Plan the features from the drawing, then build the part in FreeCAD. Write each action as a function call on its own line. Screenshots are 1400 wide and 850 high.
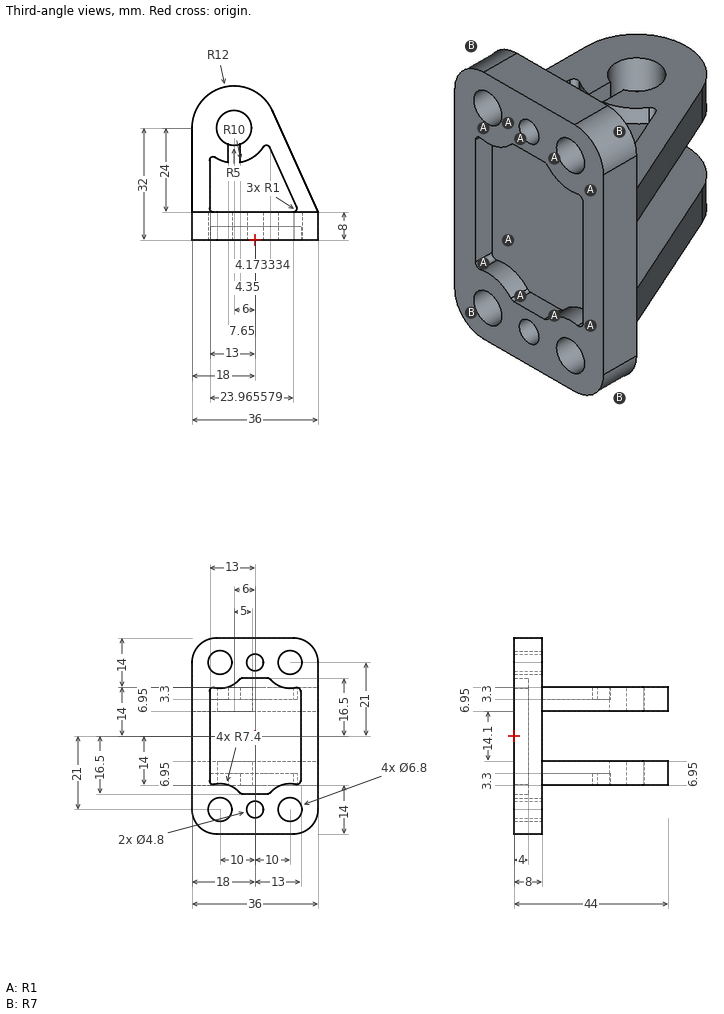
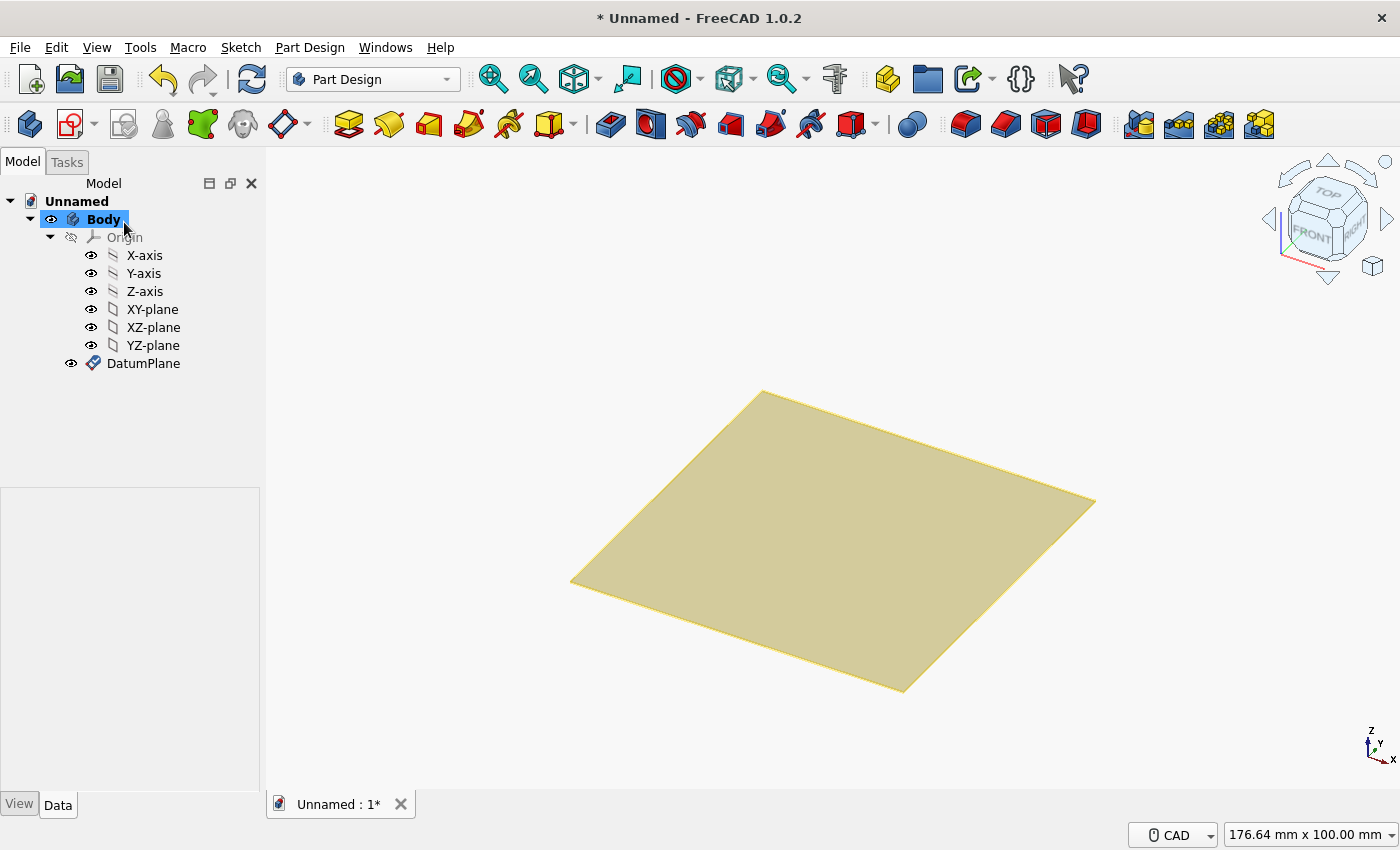
click(116, 363)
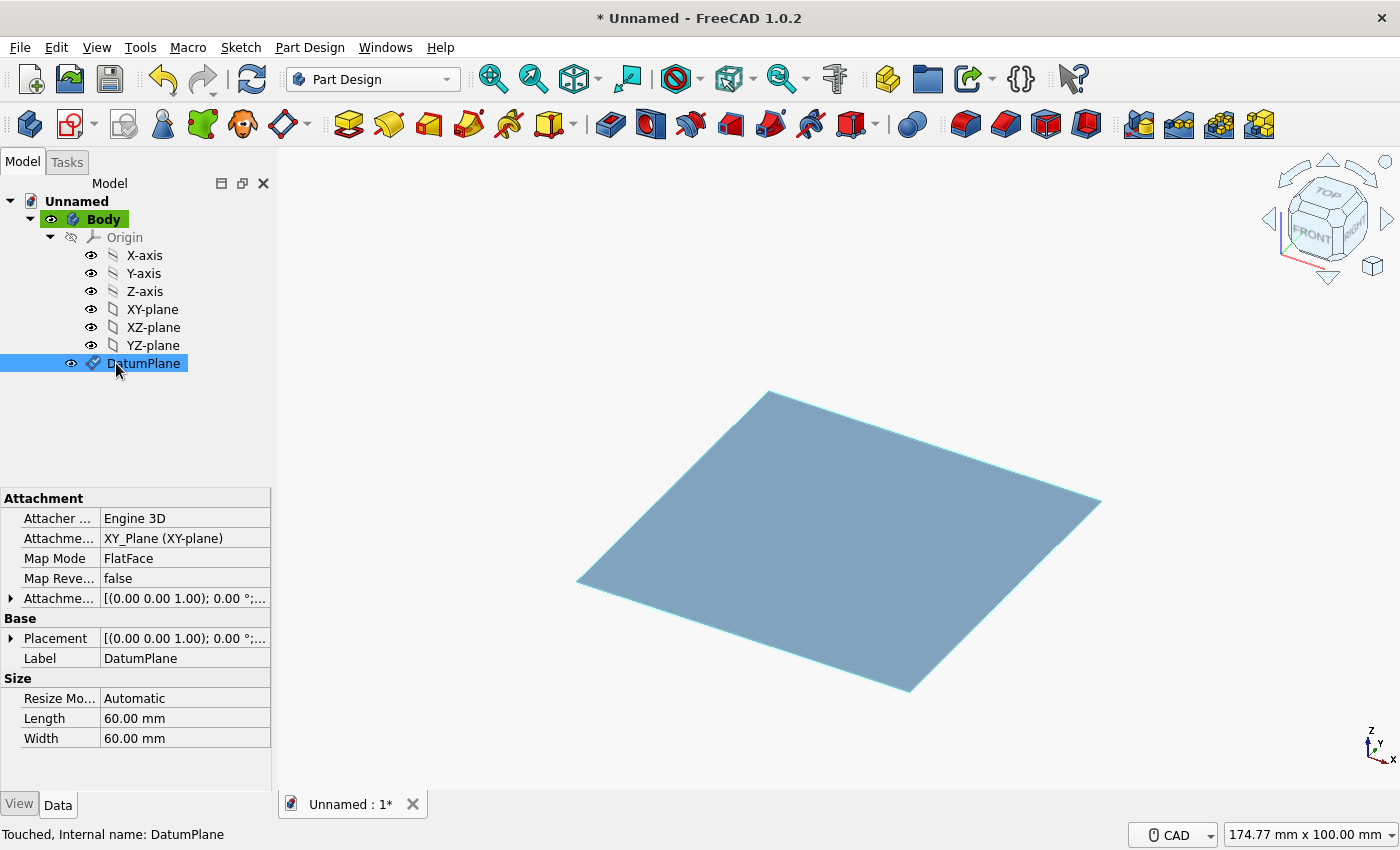
click(70, 124)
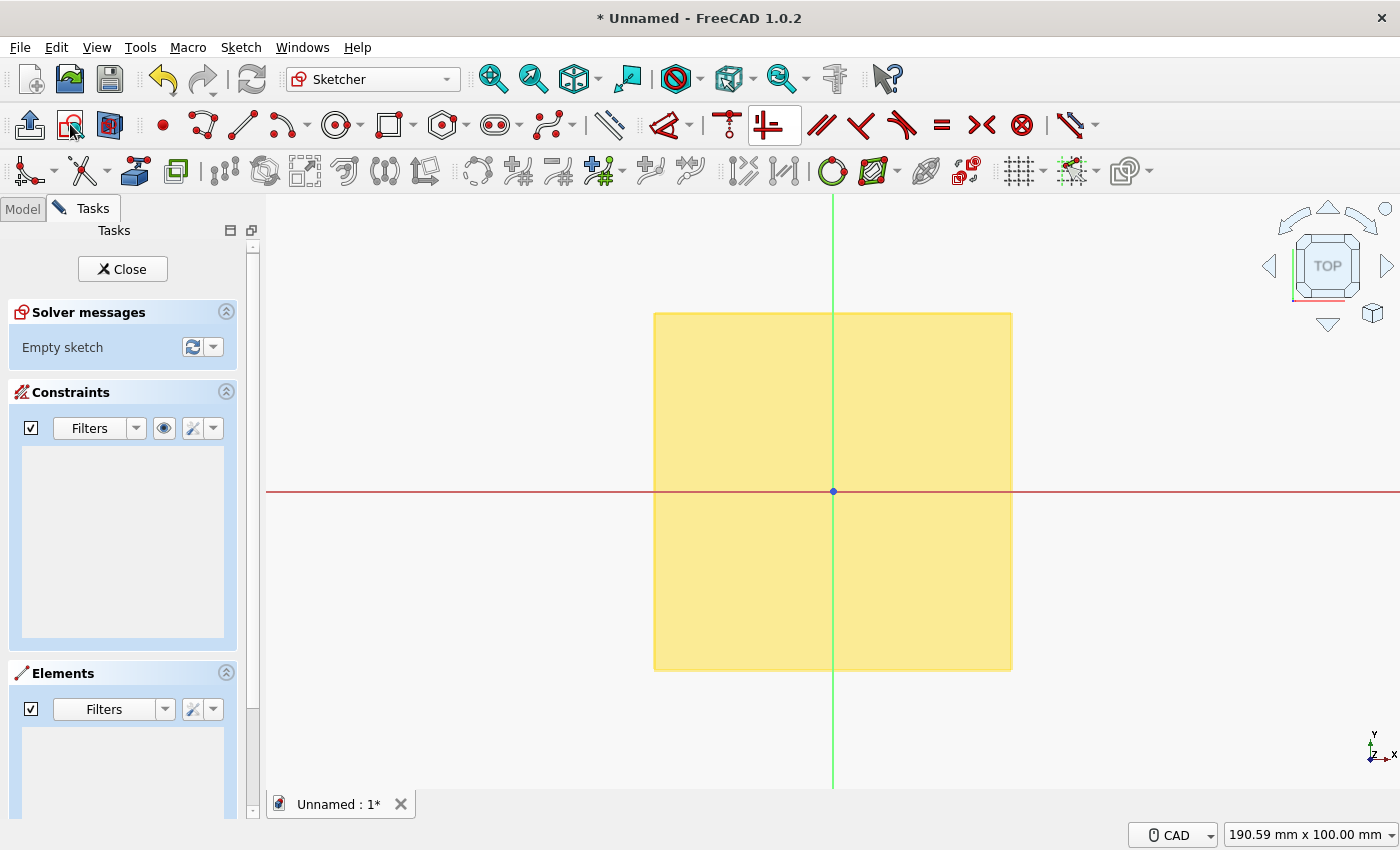
scroll(455, 761, down, 1)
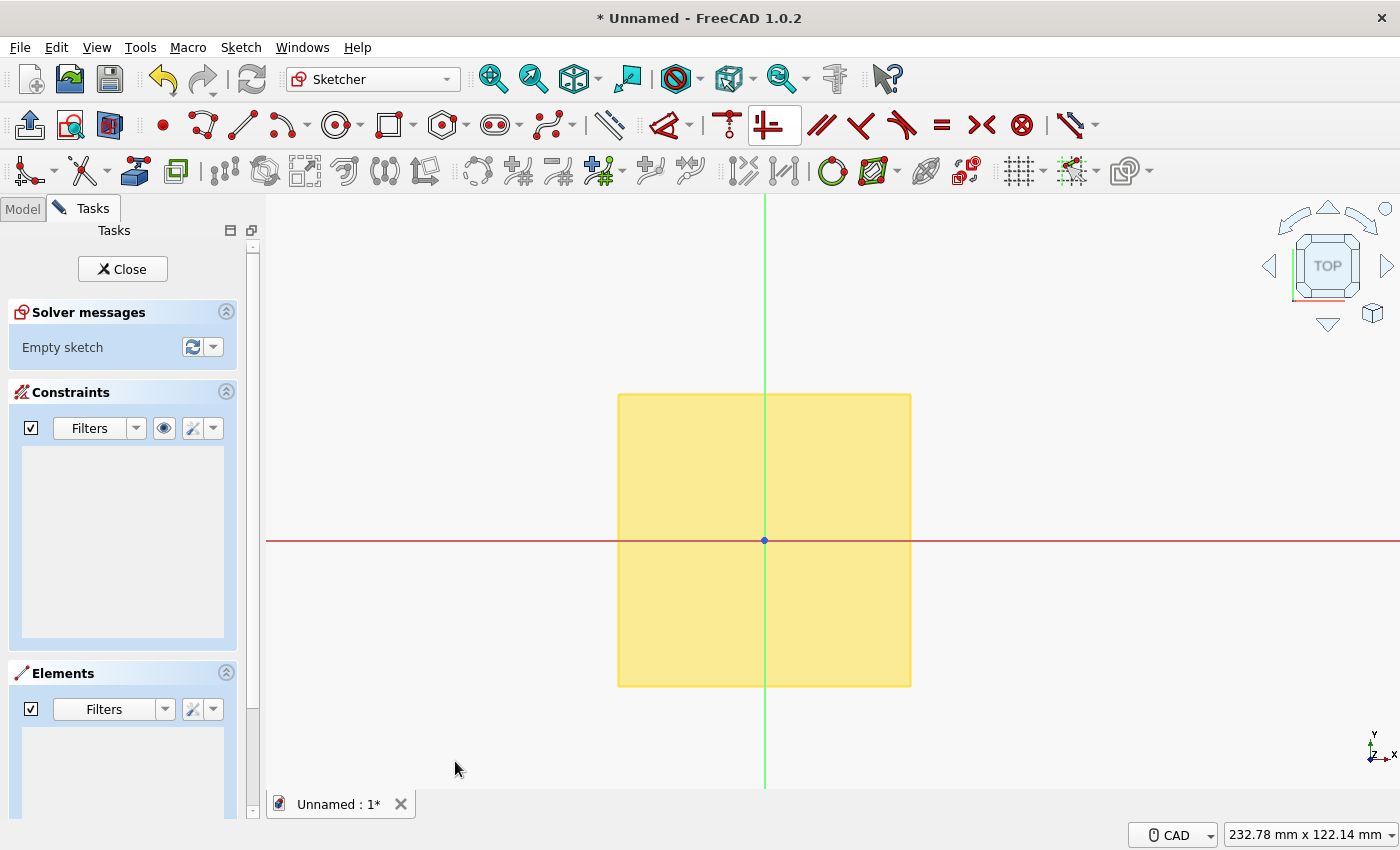
scroll(765, 364, up, 3)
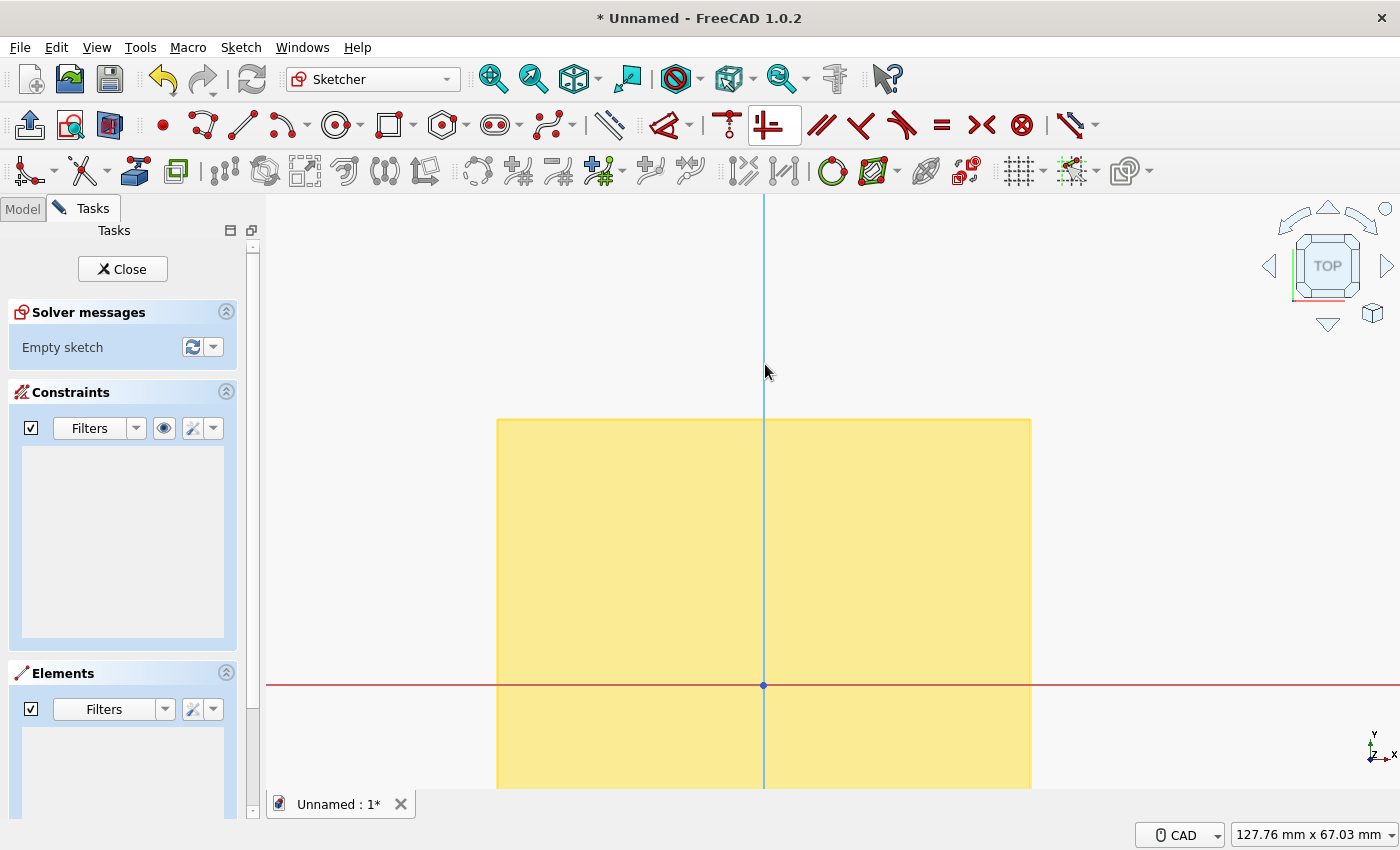
key(g)
key(m)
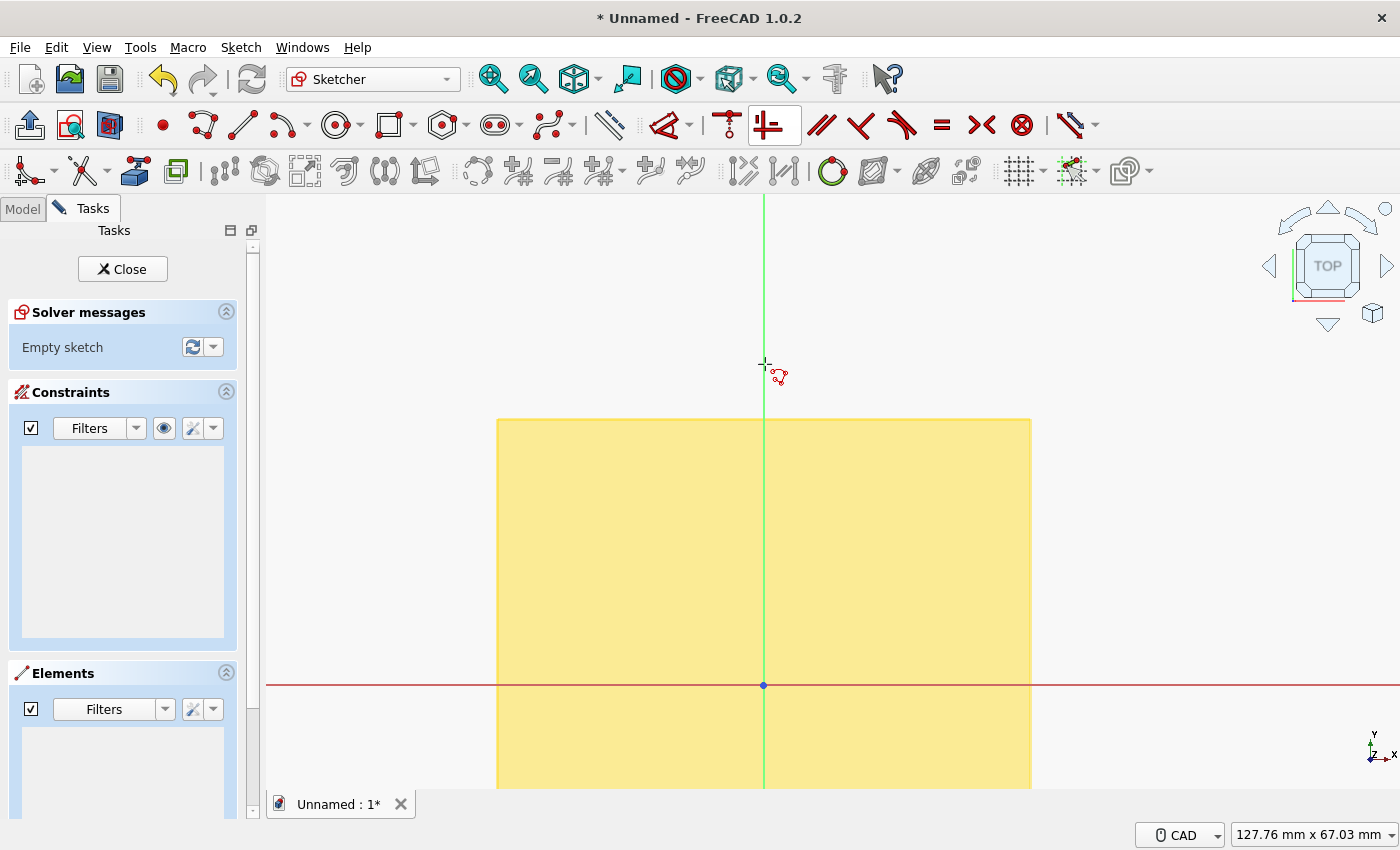
click(808, 358)
click(924, 614)
click(604, 614)
click(604, 401)
right_click(604, 401)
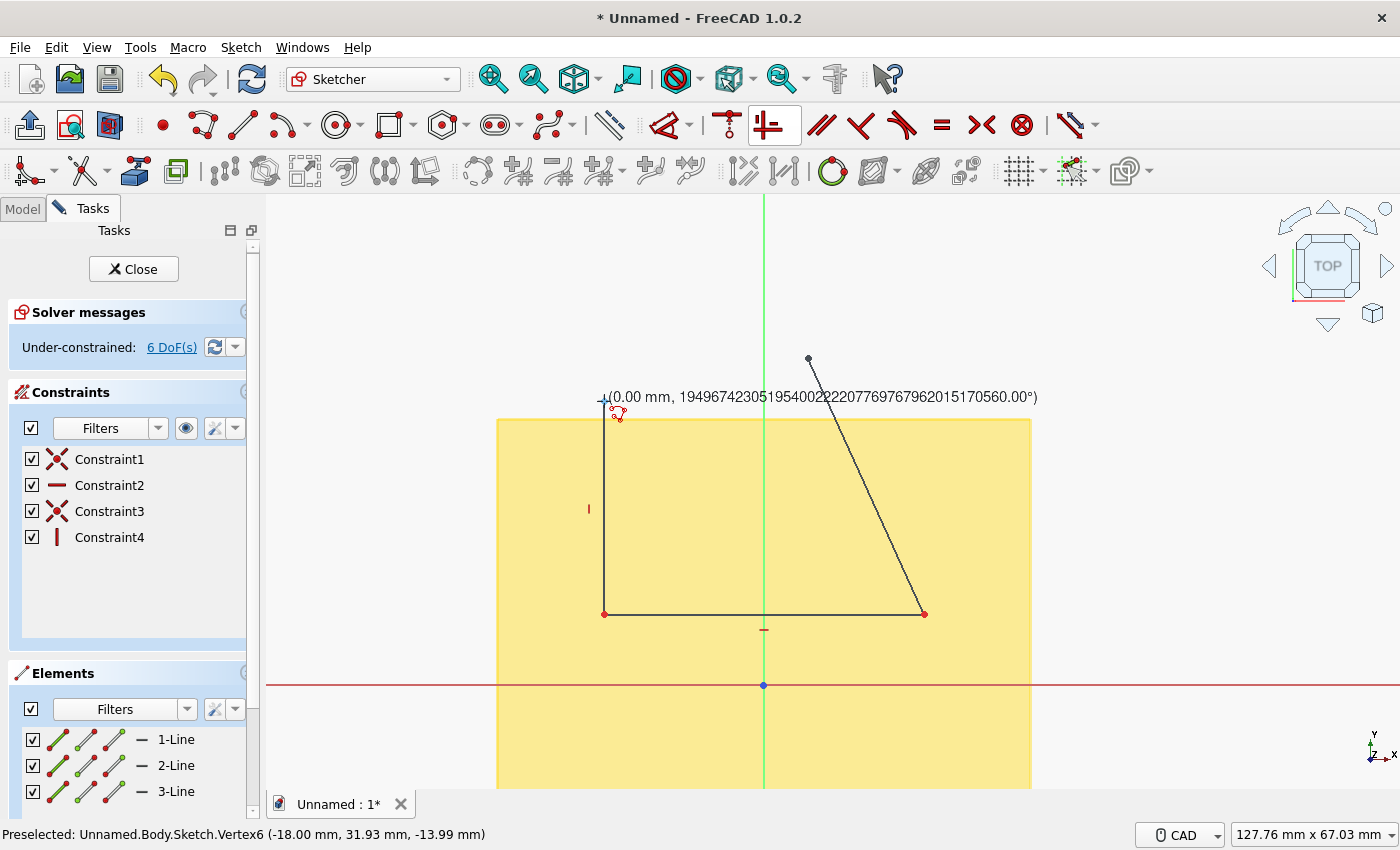
key(g)
key(3)
key(a)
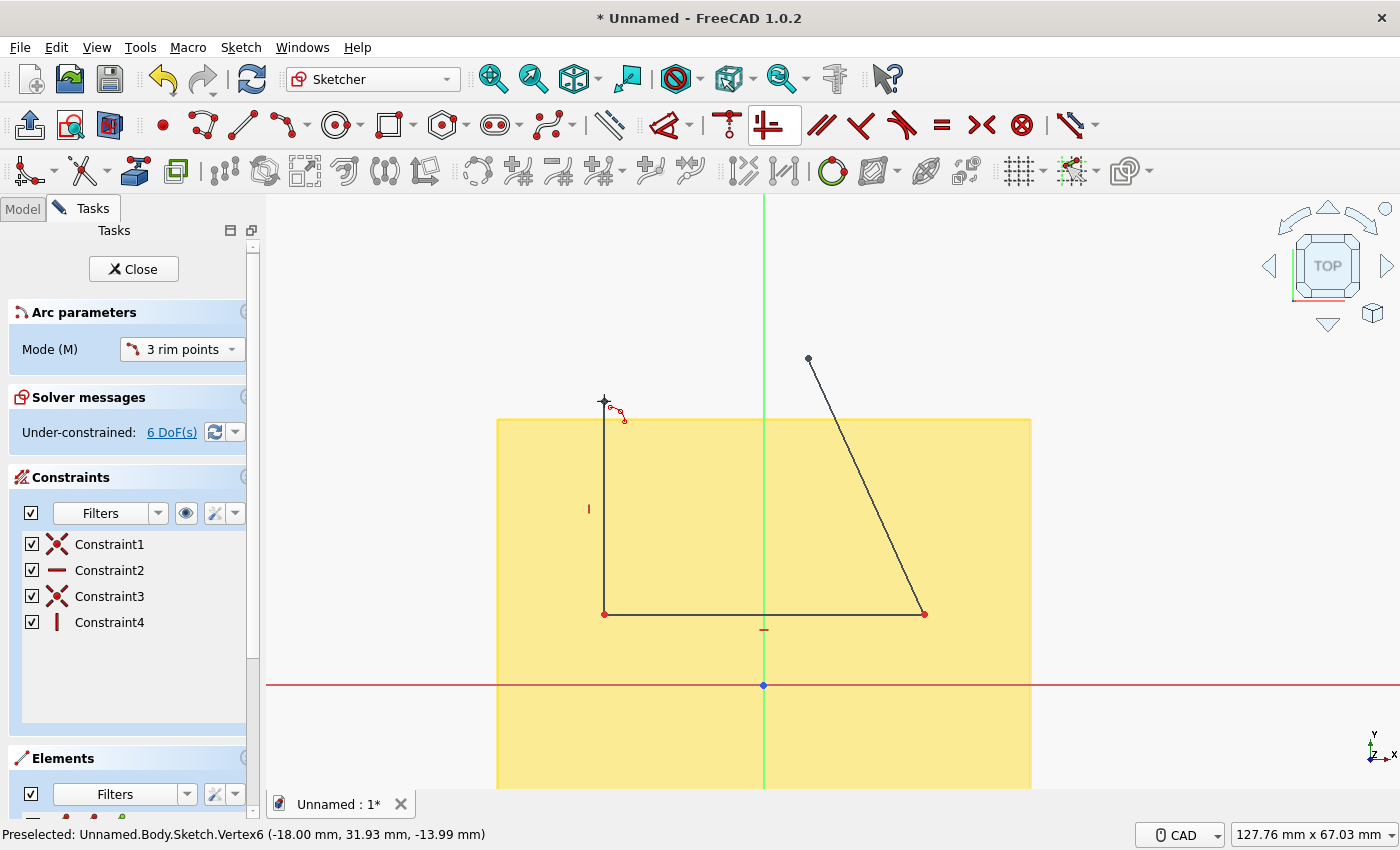
click(604, 402)
click(808, 359)
click(688, 297)
key(Escape)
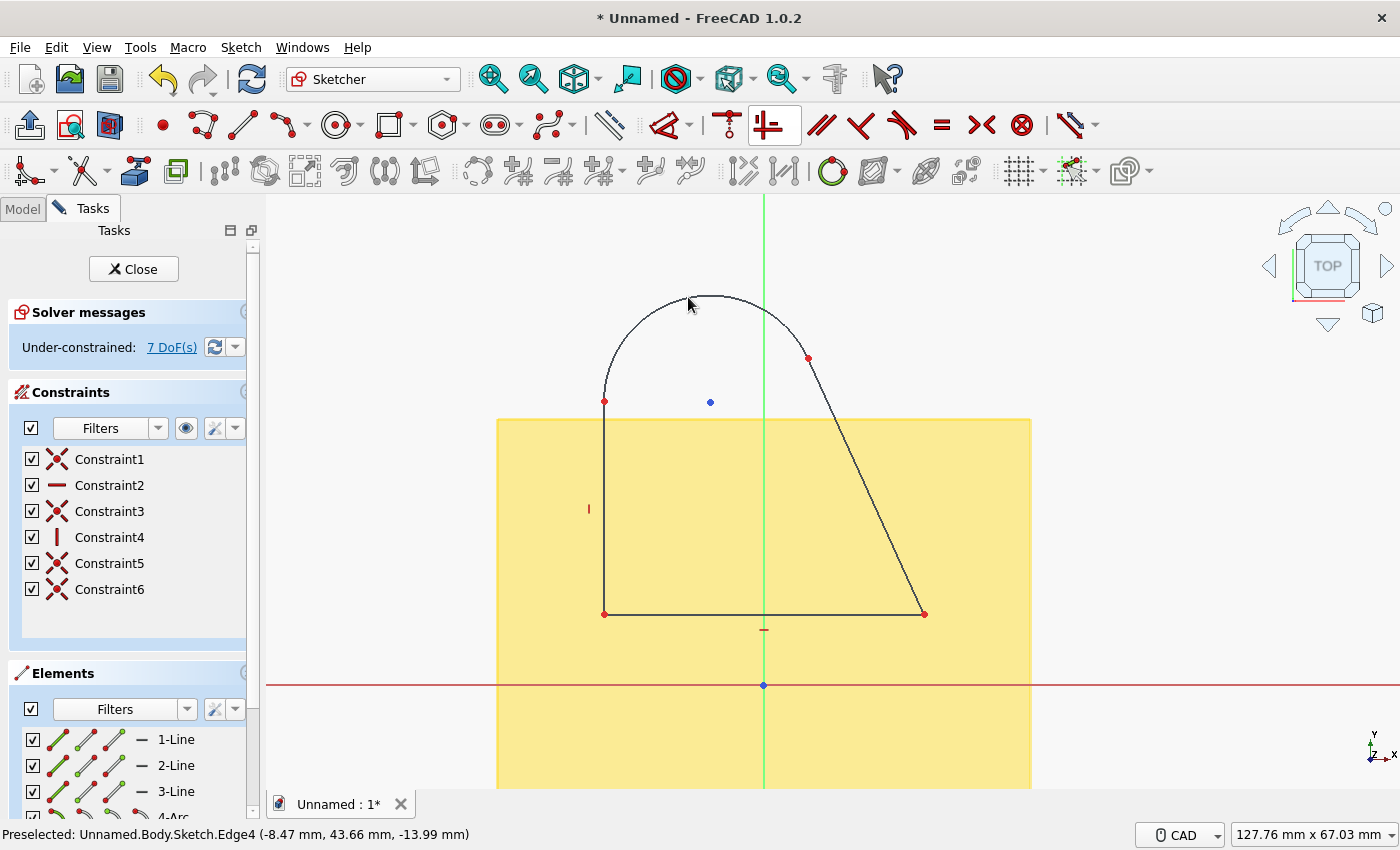
click(843, 436)